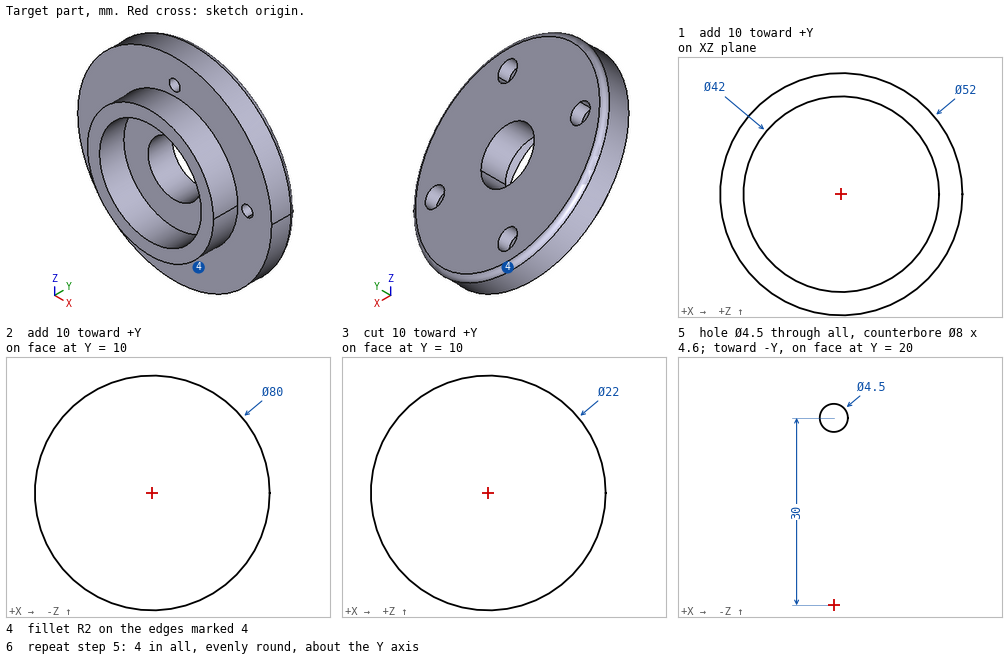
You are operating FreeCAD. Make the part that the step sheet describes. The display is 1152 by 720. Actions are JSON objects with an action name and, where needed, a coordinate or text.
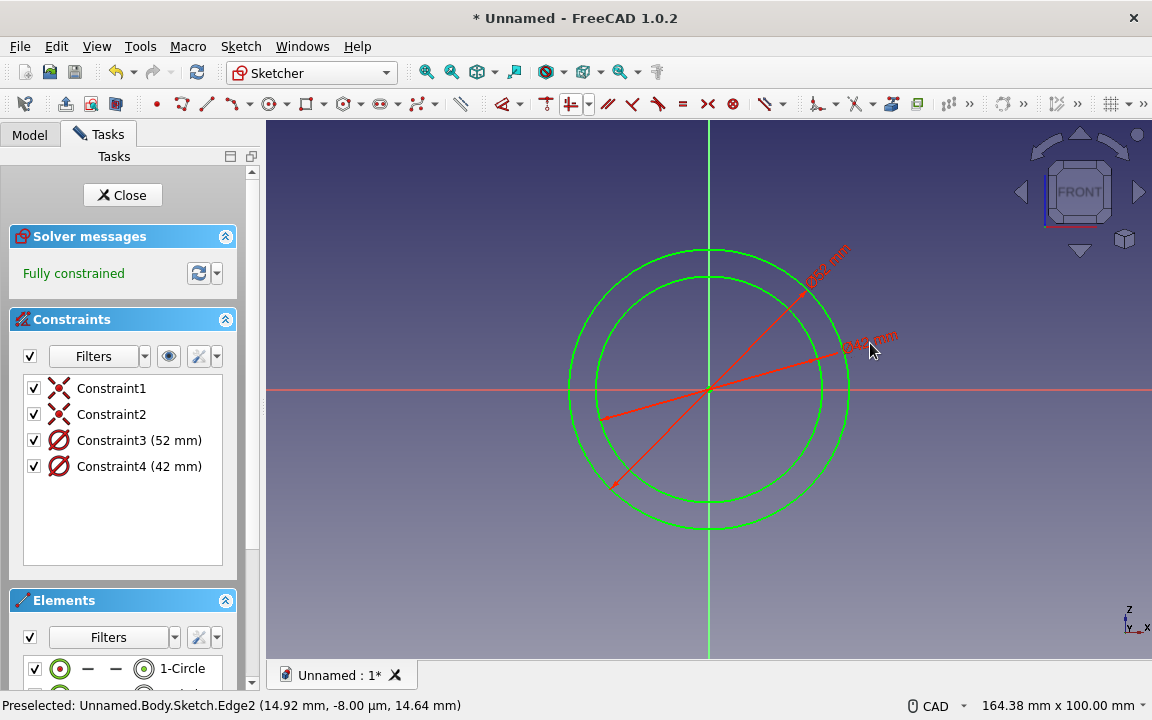
{"action": "left_click", "coordinate": [123, 195]}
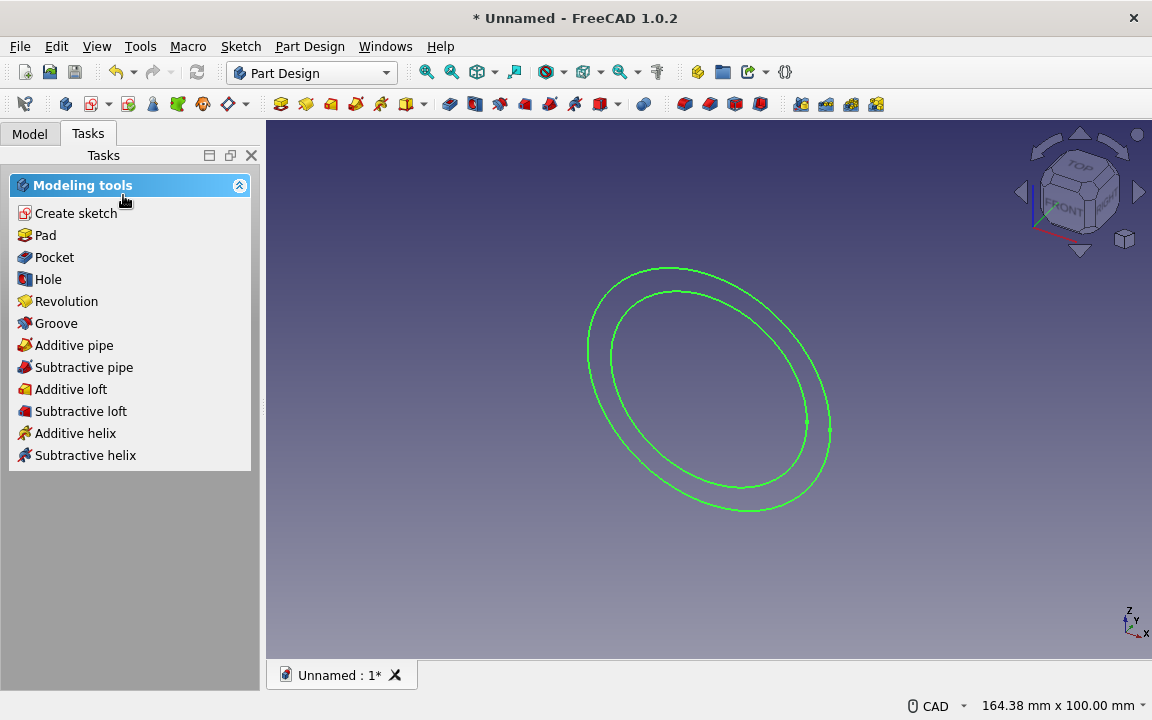
{"action": "left_click", "coordinate": [281, 104]}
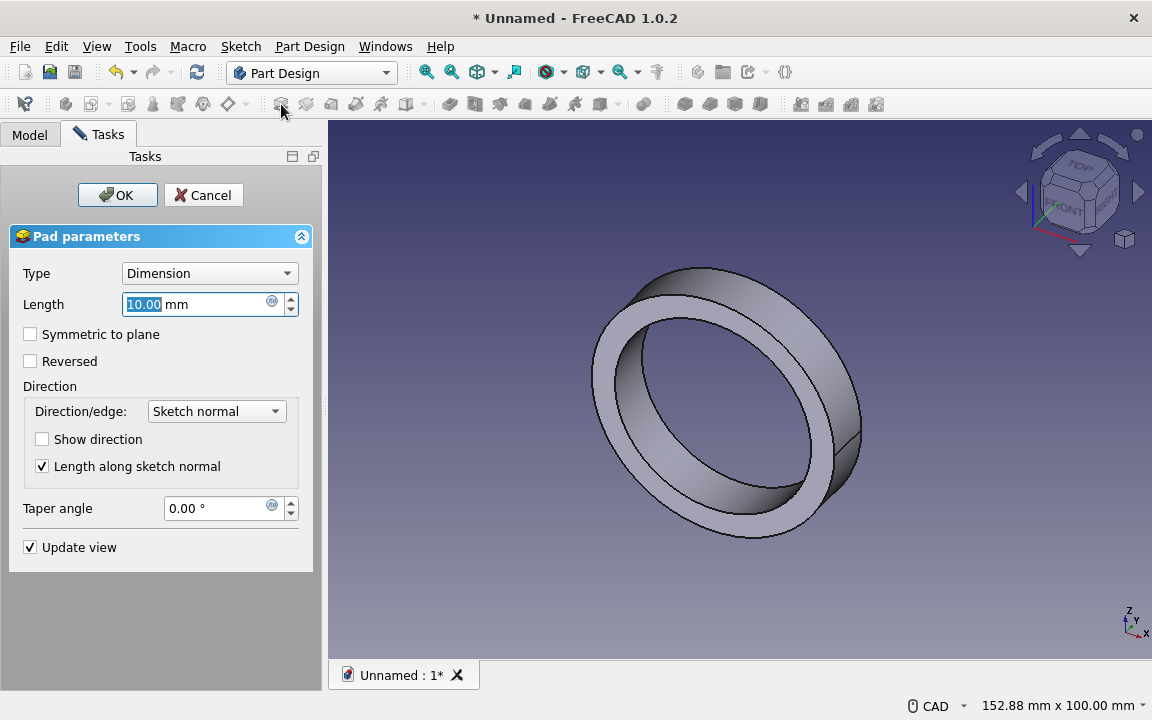
{"action": "type", "text": "10"}
{"action": "key", "text": "Tab"}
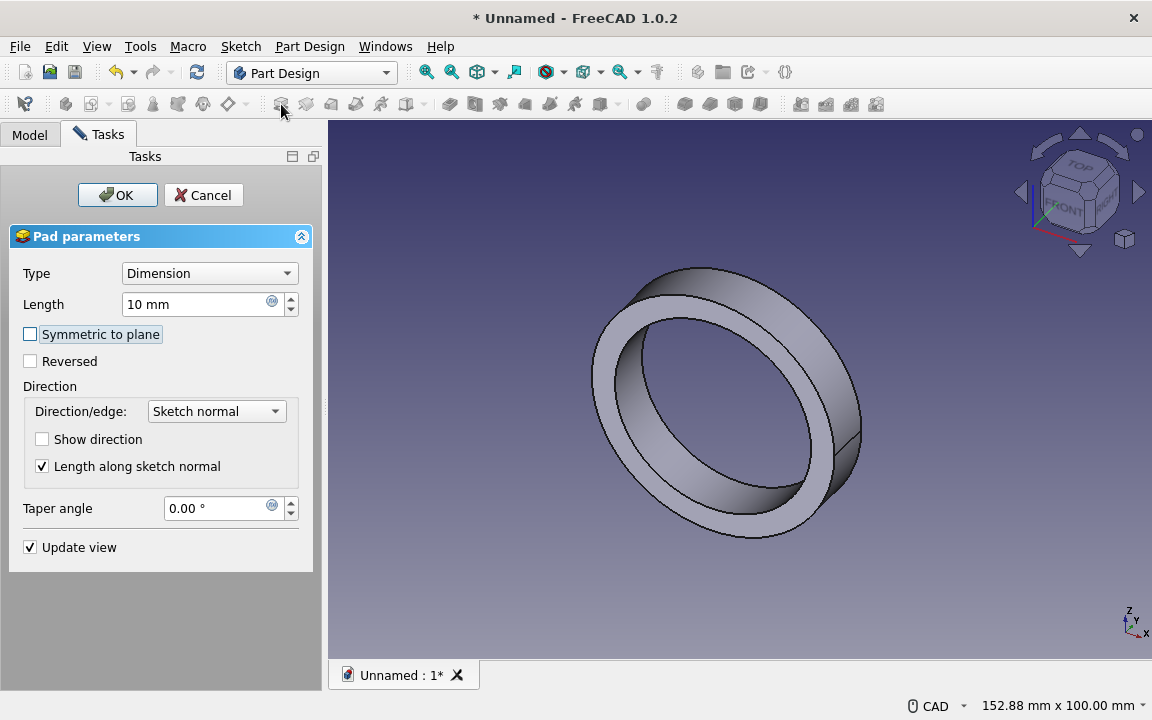
{"action": "left_click", "coordinate": [31, 361]}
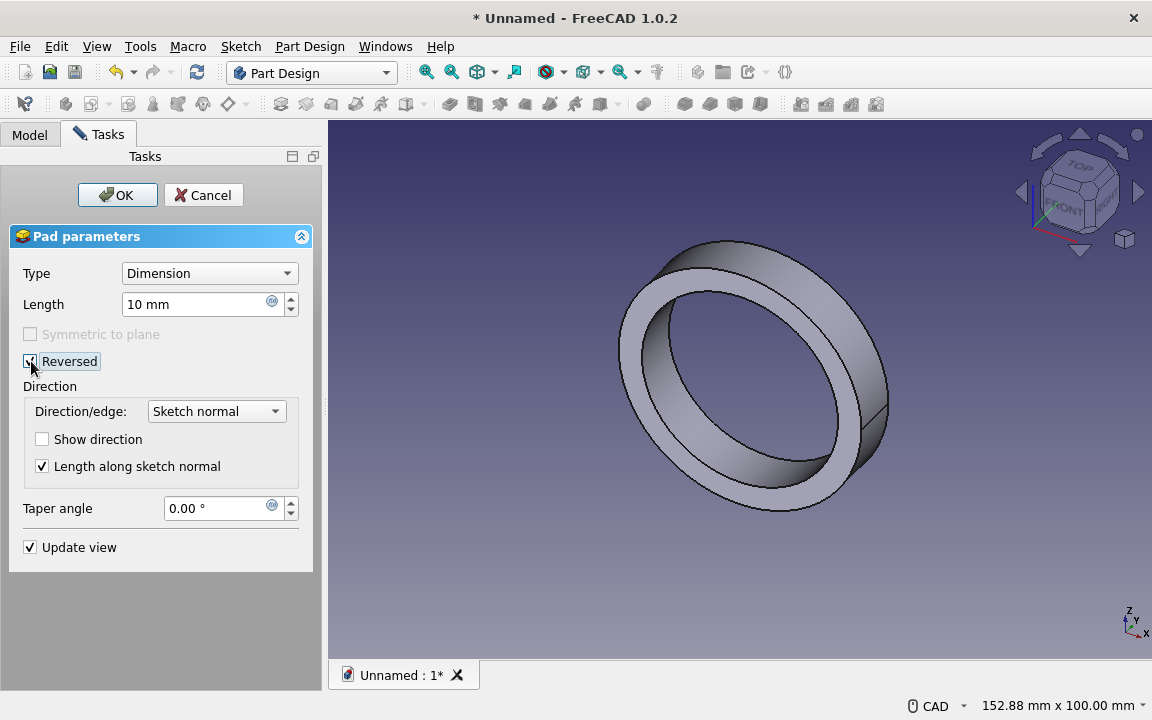
{"action": "left_click", "coordinate": [118, 195]}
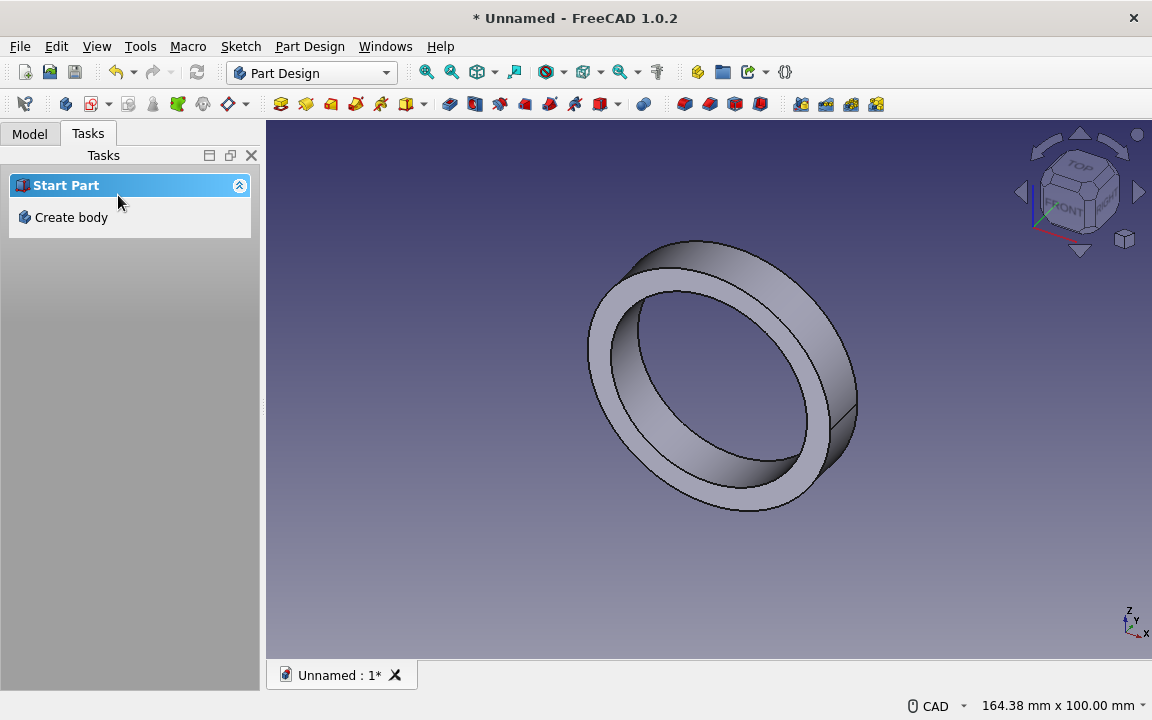
{"action": "key", "text": "4"}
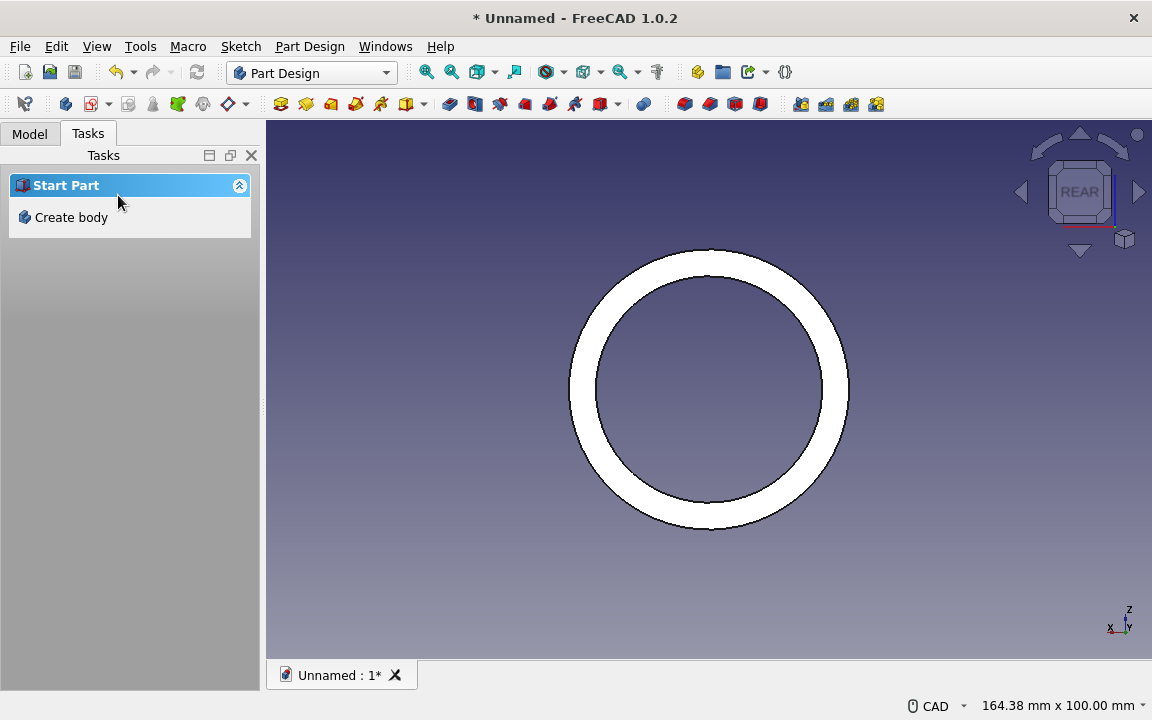
{"action": "left_click", "coordinate": [829, 348]}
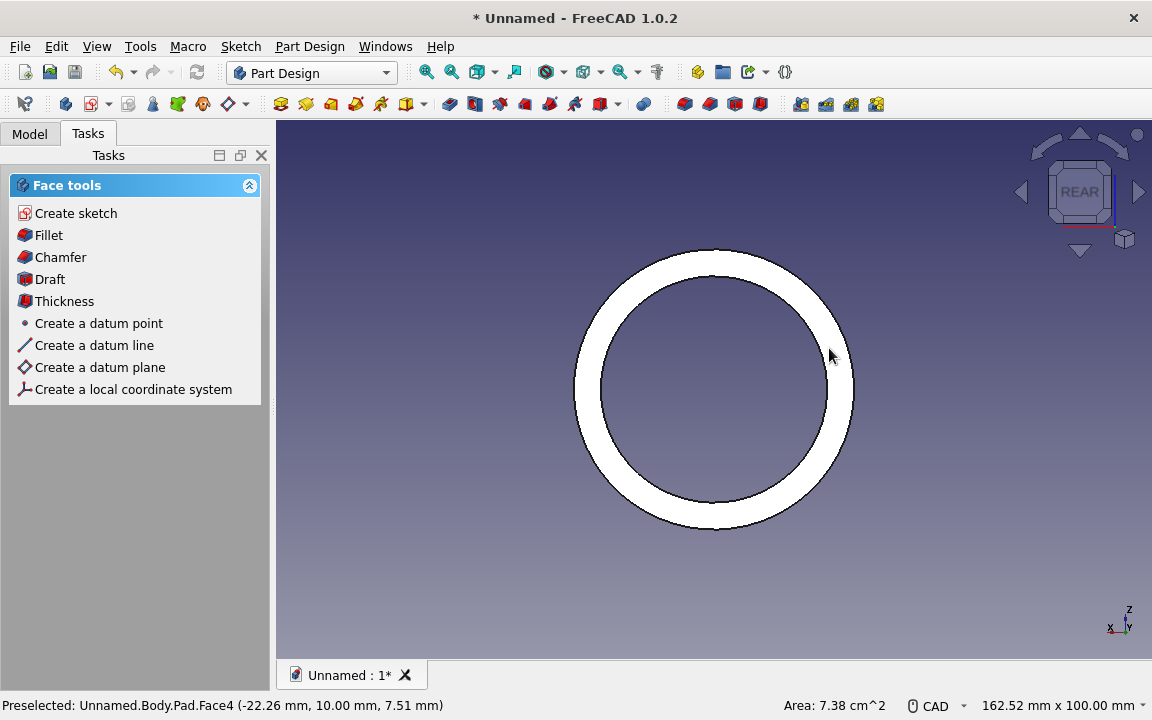
{"action": "left_click", "coordinate": [90, 104]}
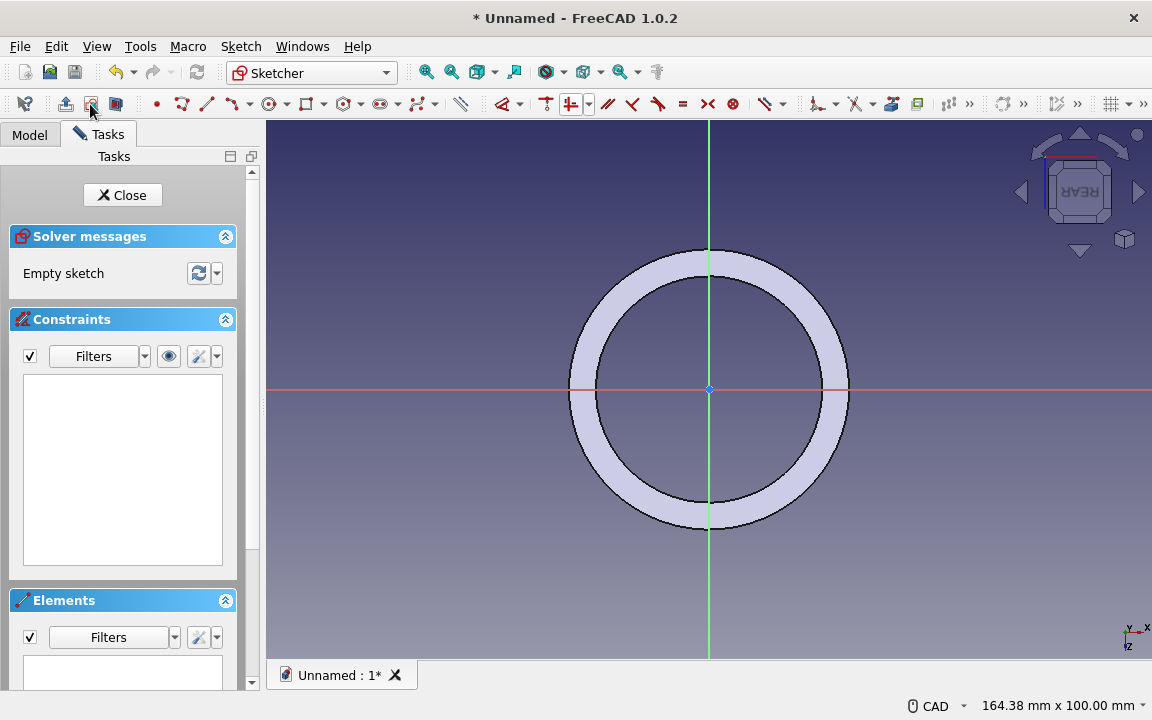
{"action": "left_click", "coordinate": [268, 104]}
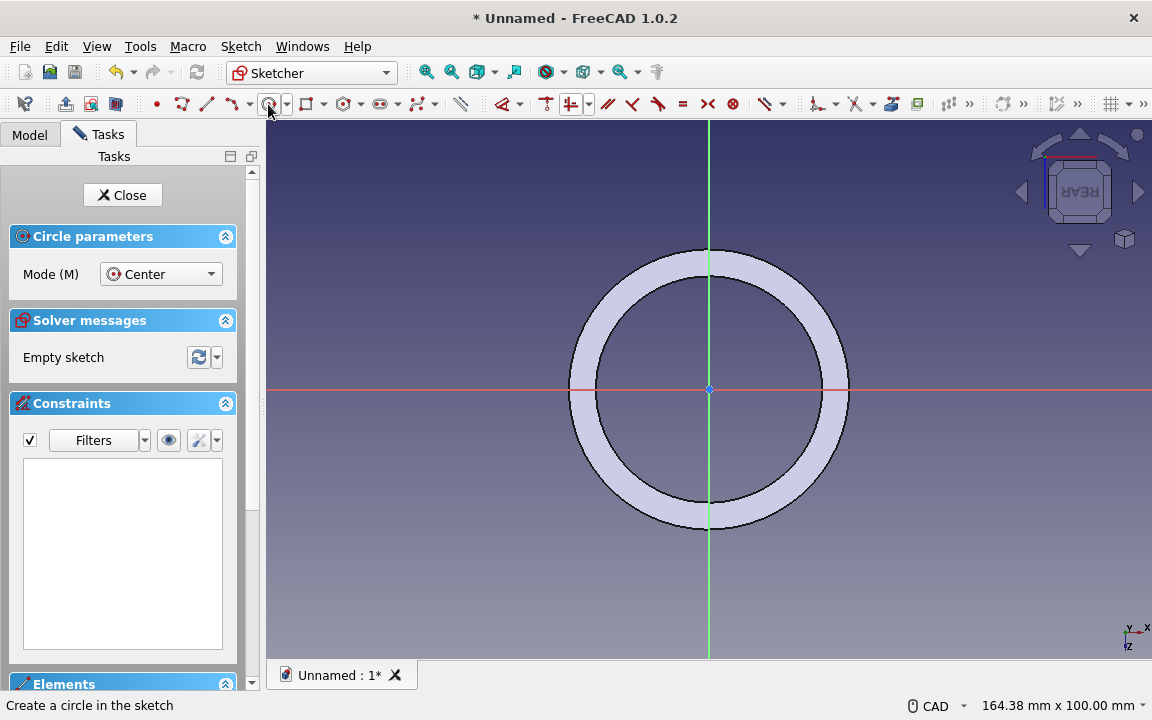
{"action": "left_click", "coordinate": [709, 390]}
{"action": "left_click", "coordinate": [861, 237]}
{"action": "key", "text": "Escape"}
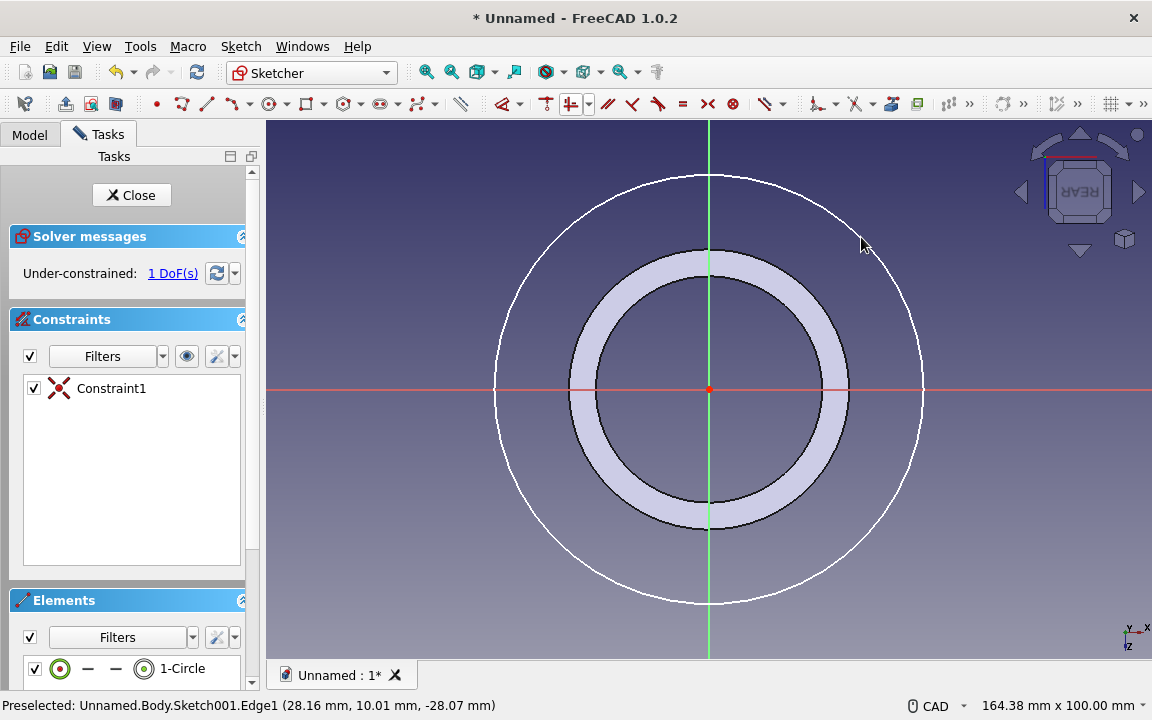
{"action": "left_click", "coordinate": [502, 104]}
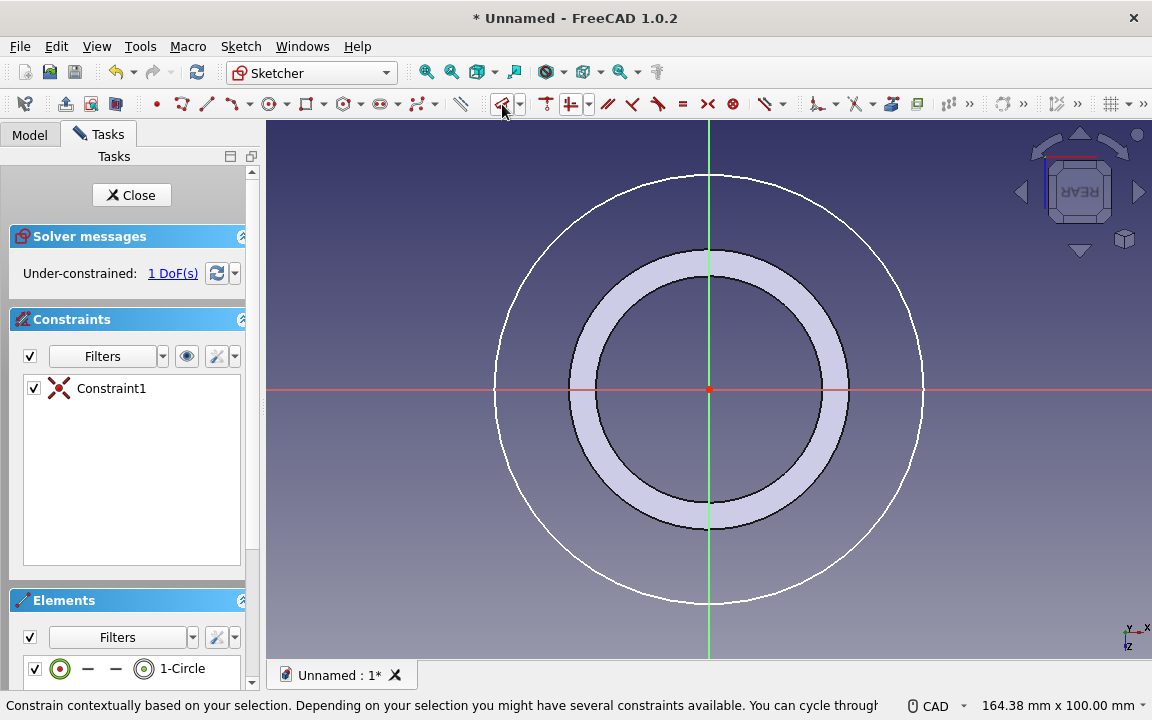
{"action": "left_click", "coordinate": [860, 237]}
{"action": "left_click", "coordinate": [883, 214]}